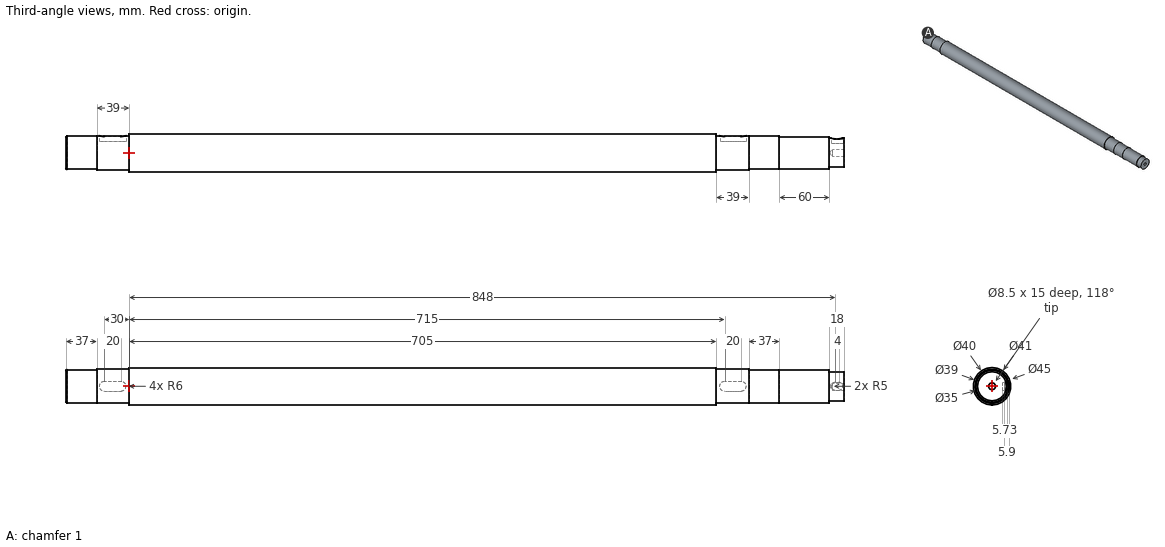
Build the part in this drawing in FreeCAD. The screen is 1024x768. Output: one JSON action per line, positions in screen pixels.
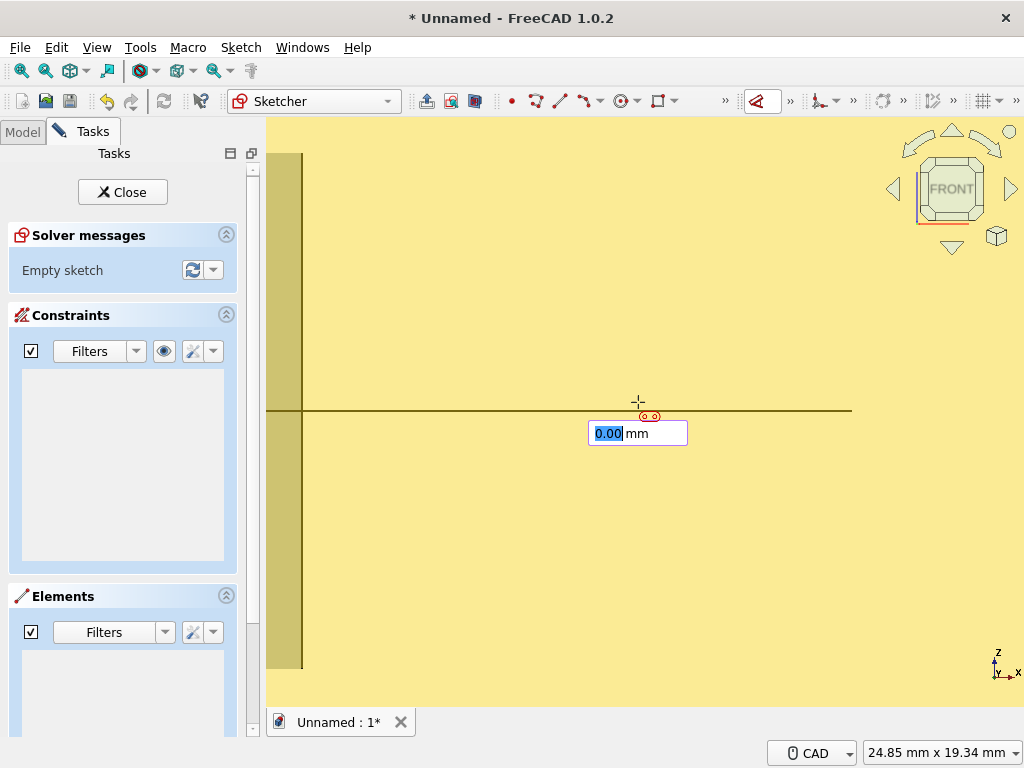
{"action": "left_click", "coordinate": [577, 563]}
{"action": "key", "text": "Escape"}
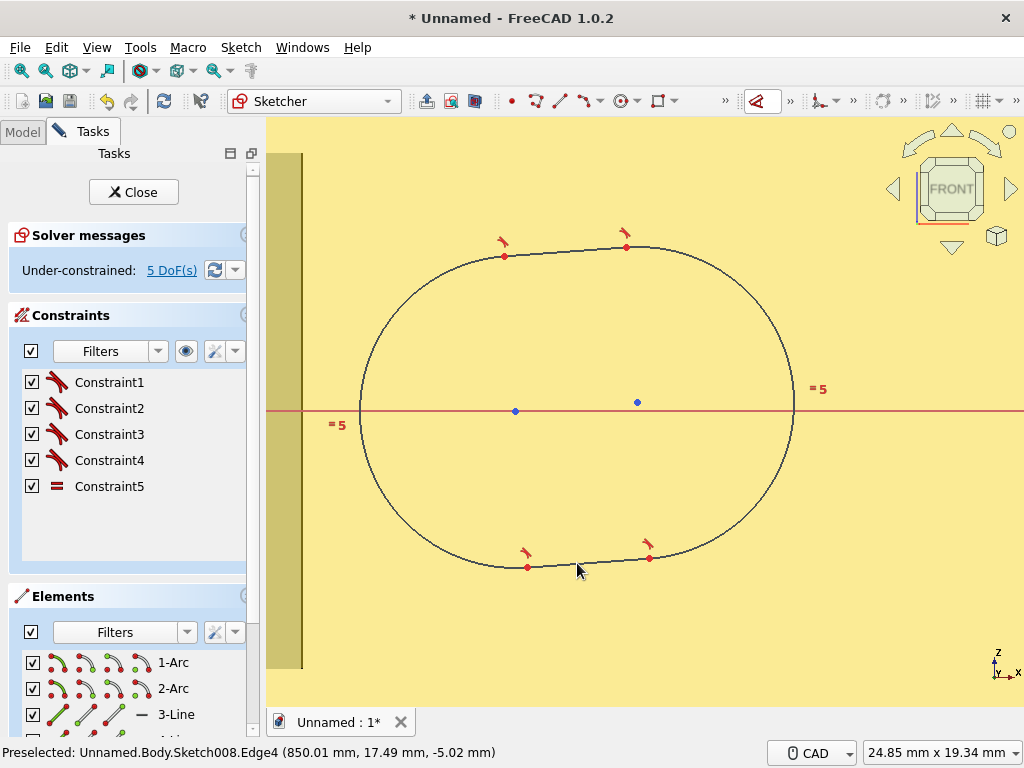
{"action": "left_click", "coordinate": [541, 254]}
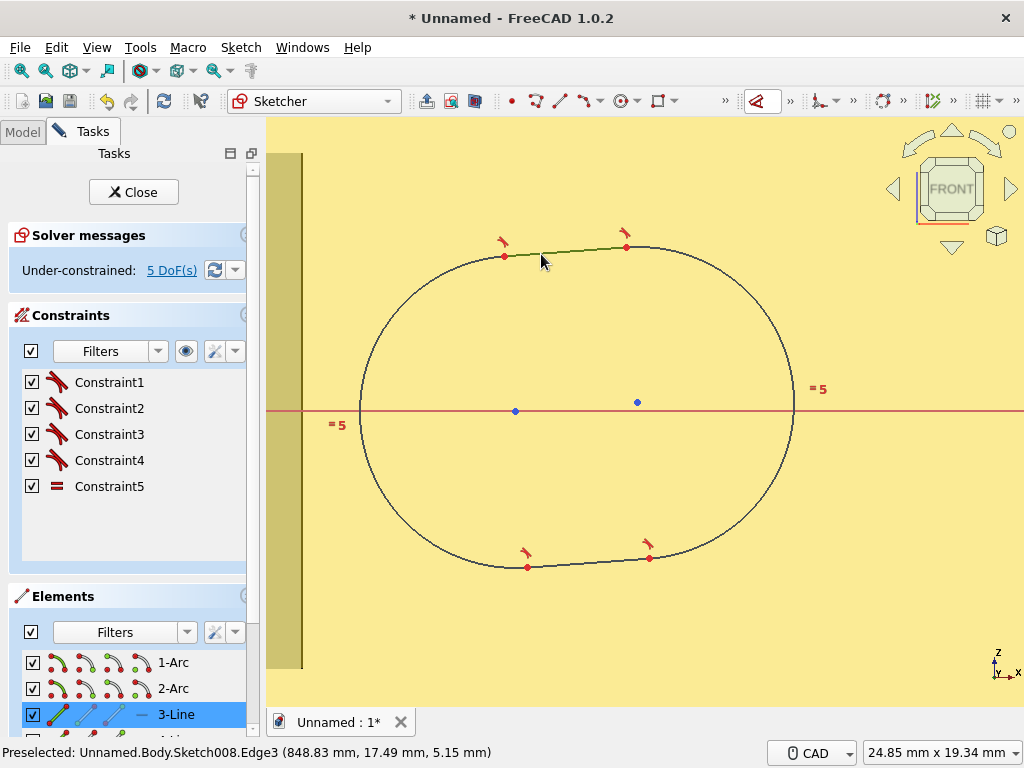
{"action": "key", "text": "h"}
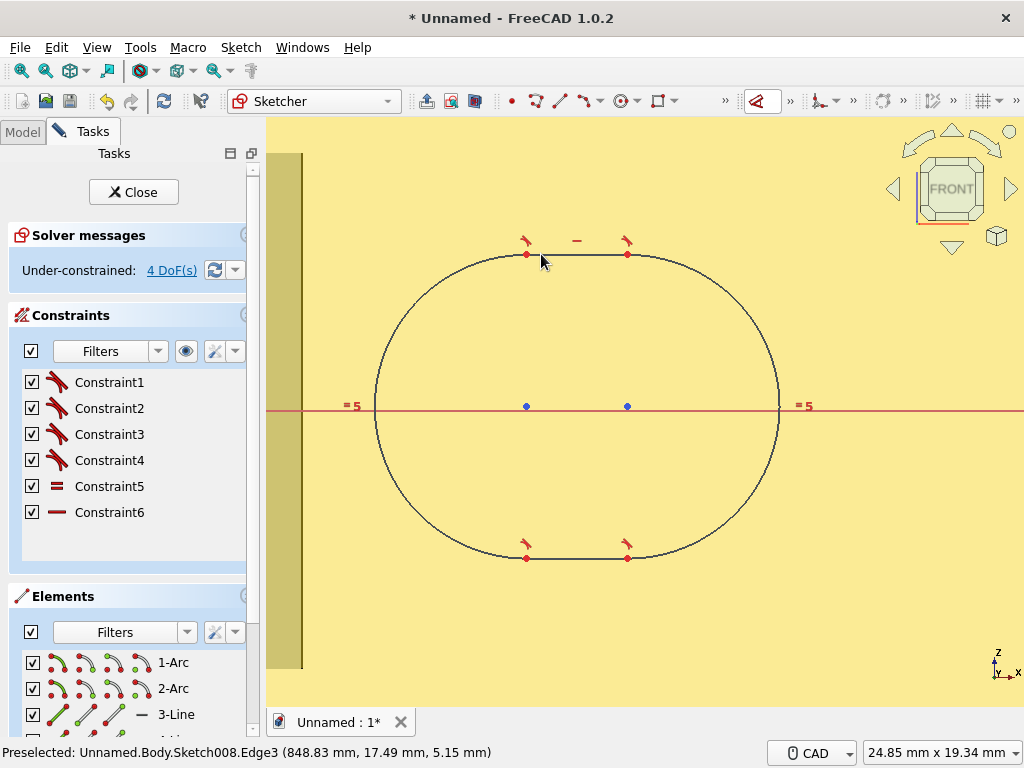
{"action": "left_click", "coordinate": [527, 407]}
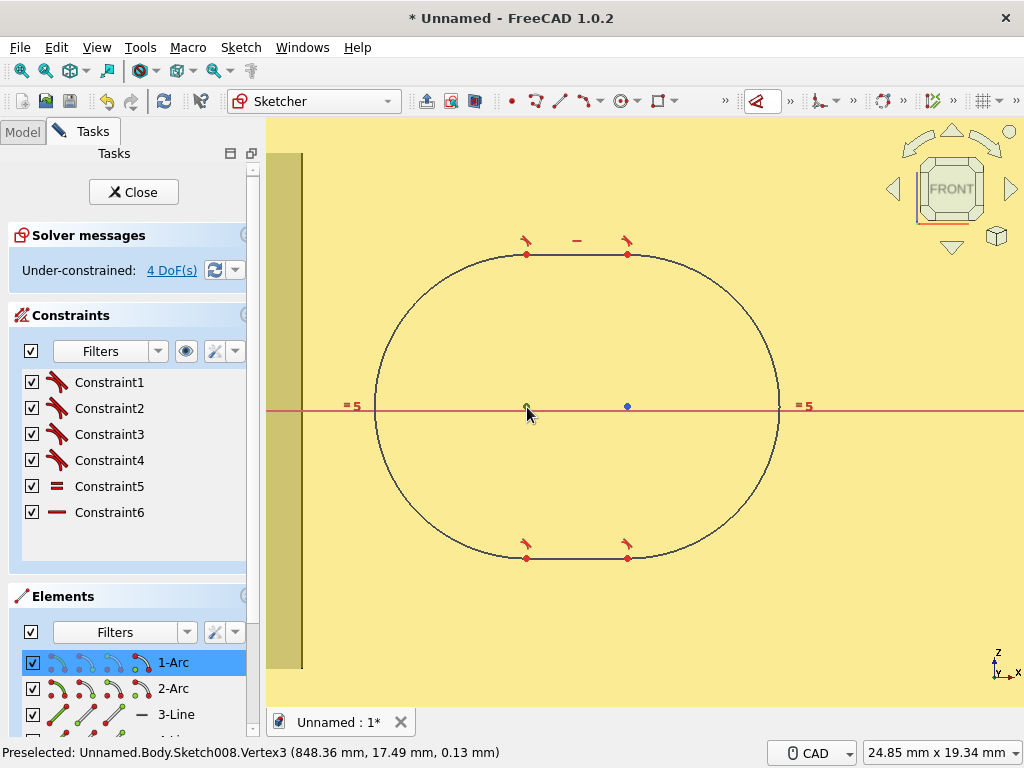
{"action": "left_click", "coordinate": [334, 411]}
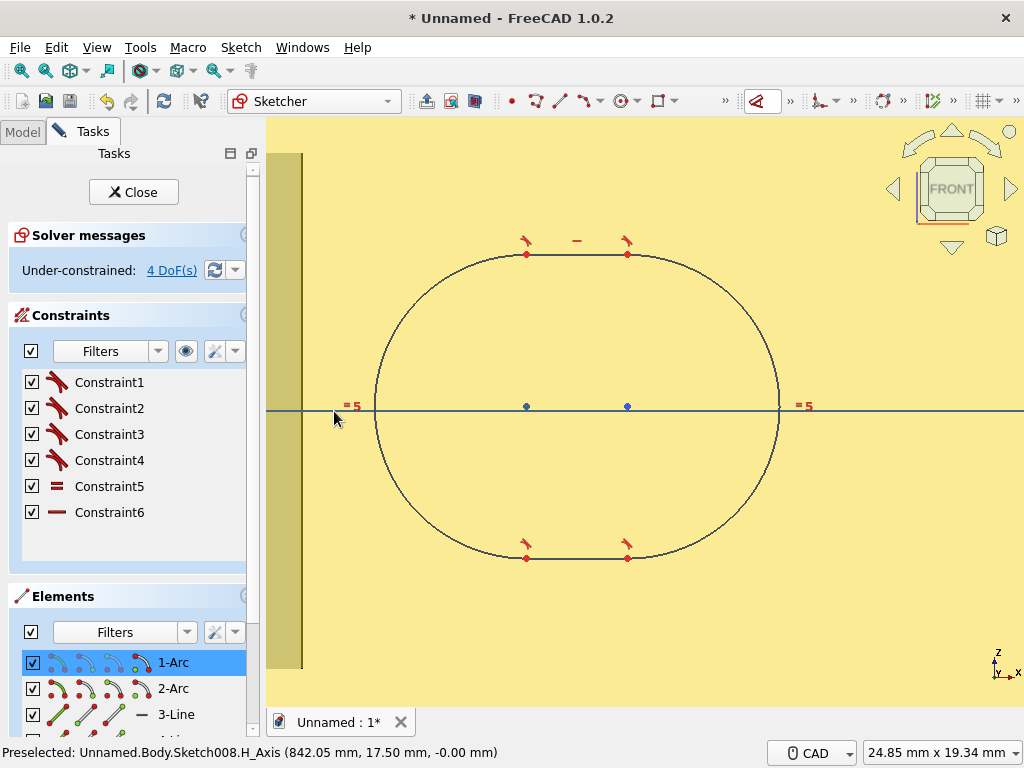
{"action": "key", "text": "c"}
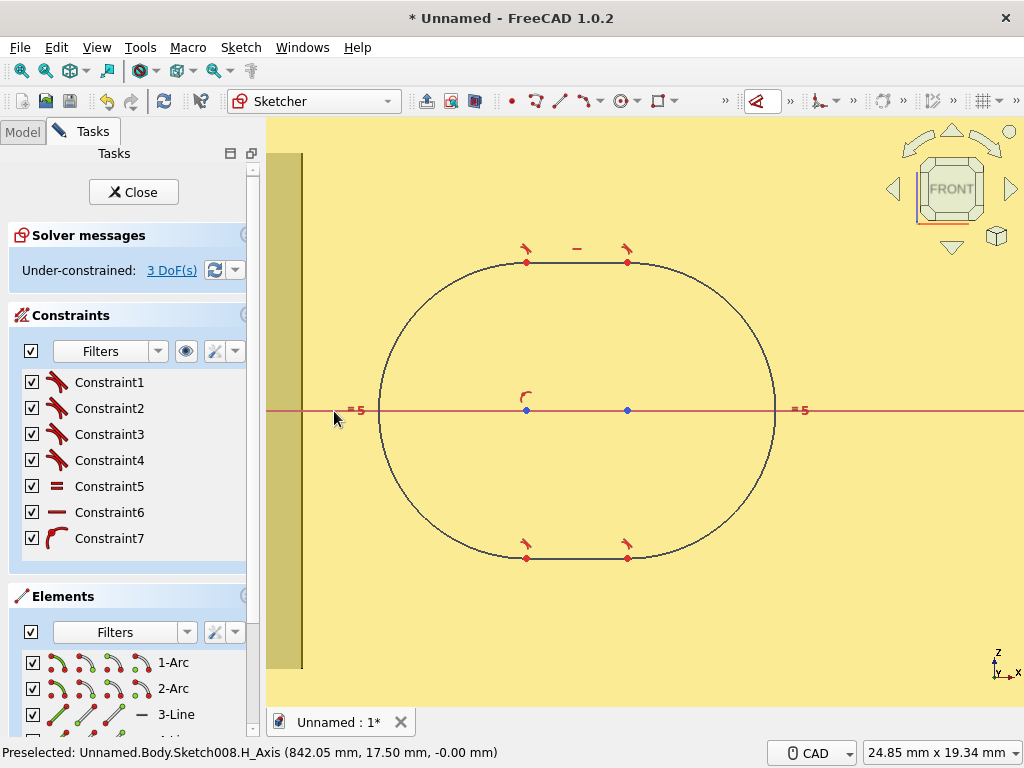
{"action": "left_click", "coordinate": [407, 324]}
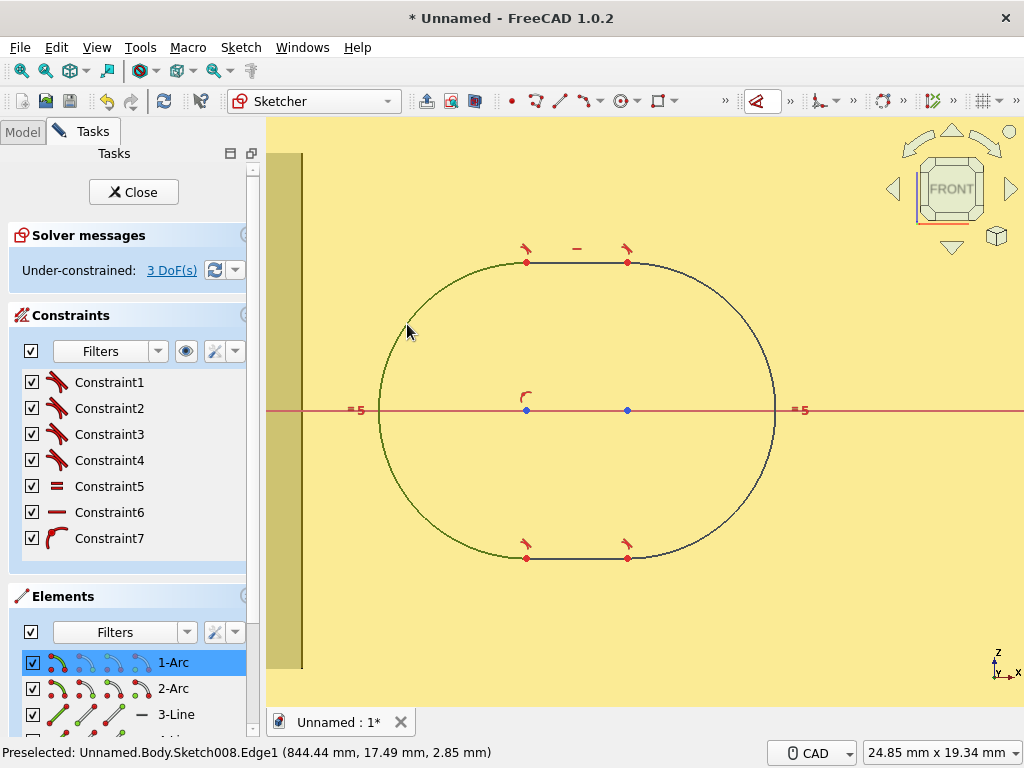
{"action": "key", "text": "k r"}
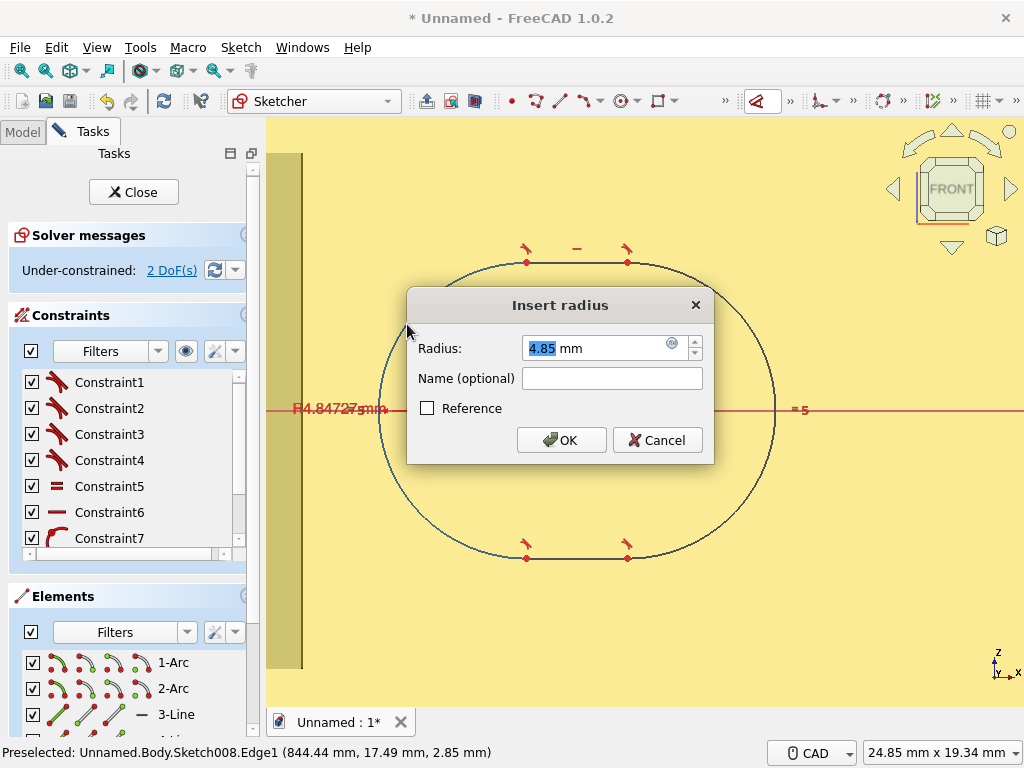
{"action": "type", "text": "5"}
{"action": "key", "text": "Return"}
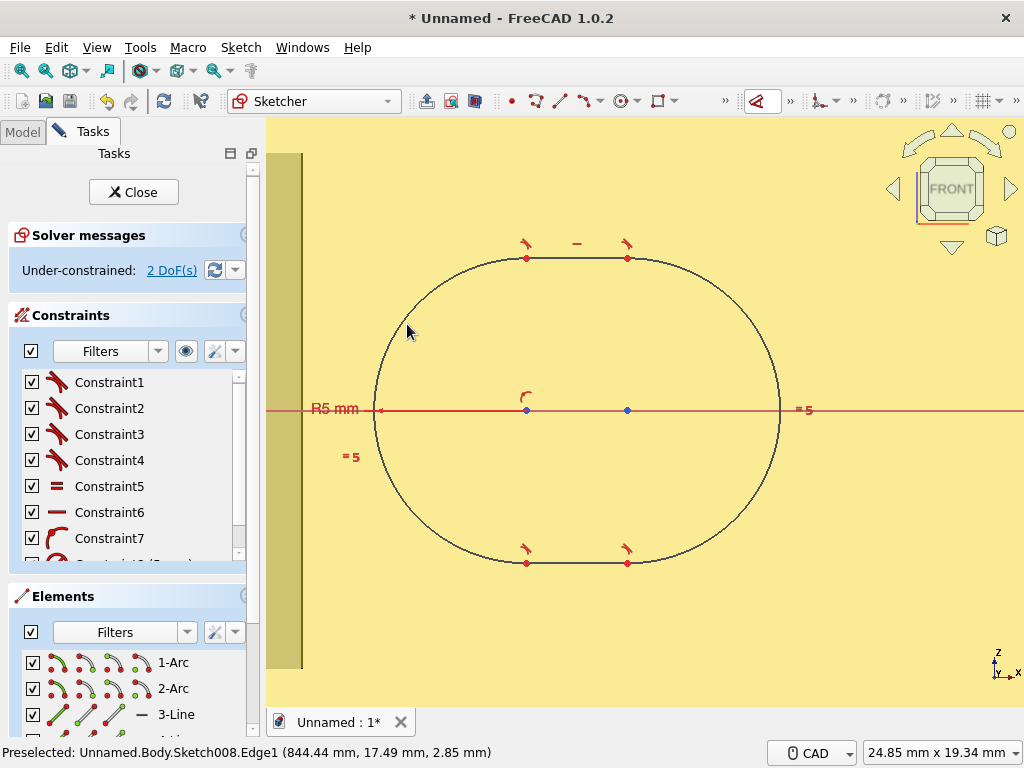
{"action": "left_click", "coordinate": [557, 258]}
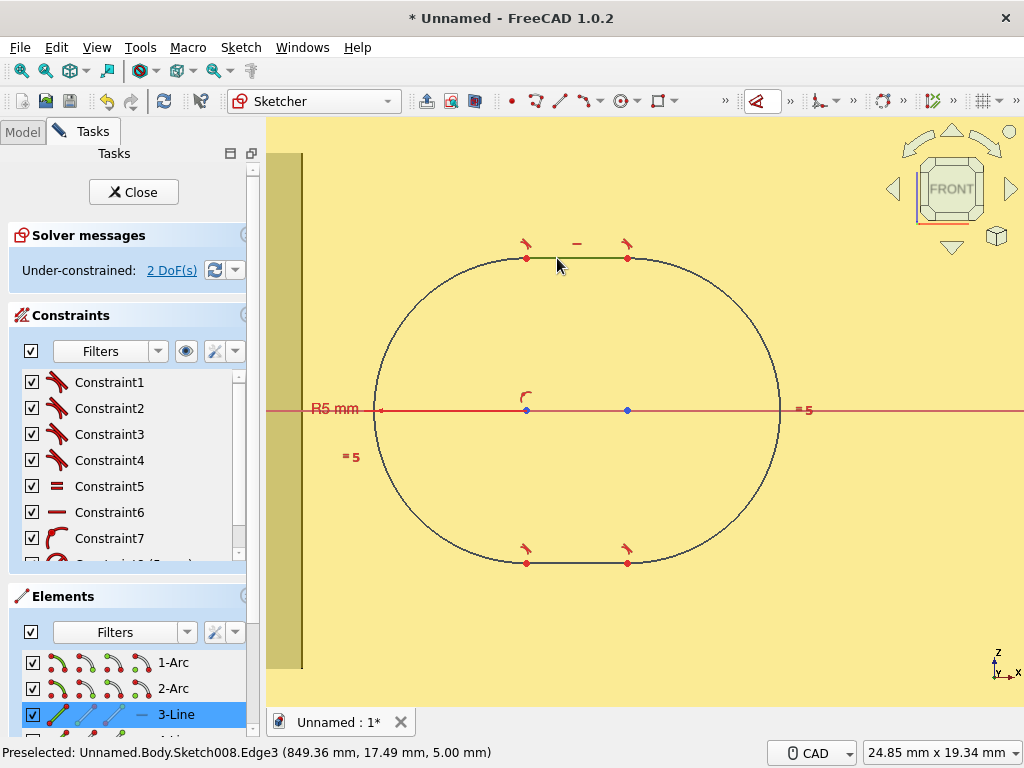
{"action": "left_click", "coordinate": [776, 102]}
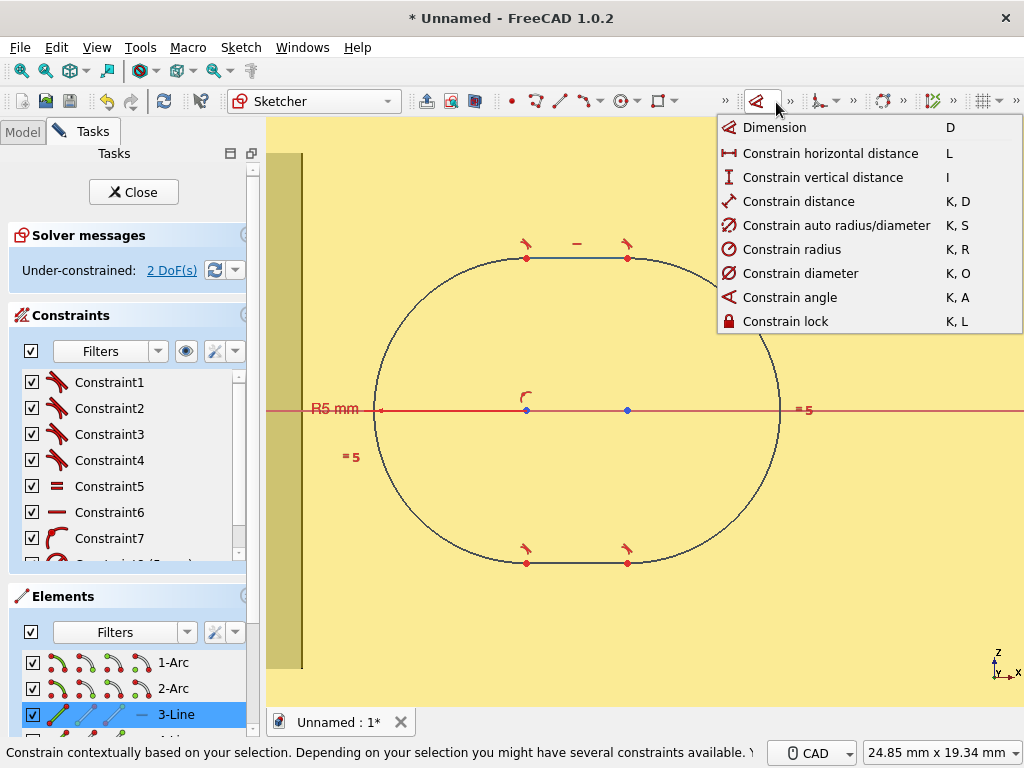
{"action": "left_click", "coordinate": [870, 153]}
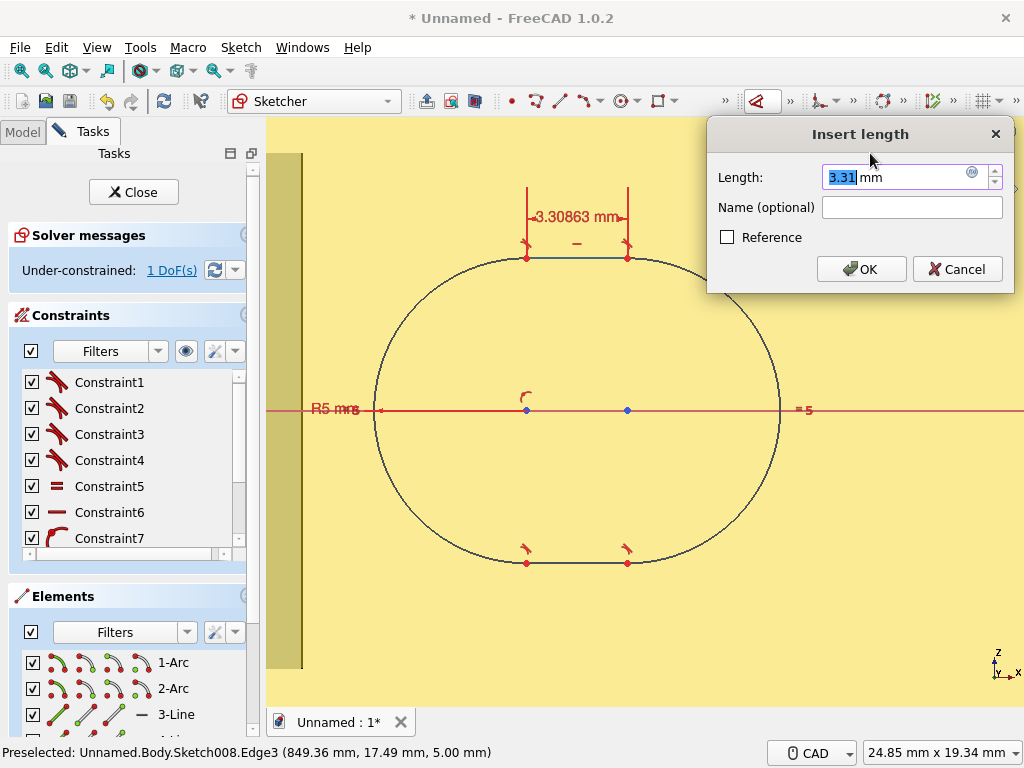
{"action": "type", "text": "4"}
{"action": "key", "text": "Return"}